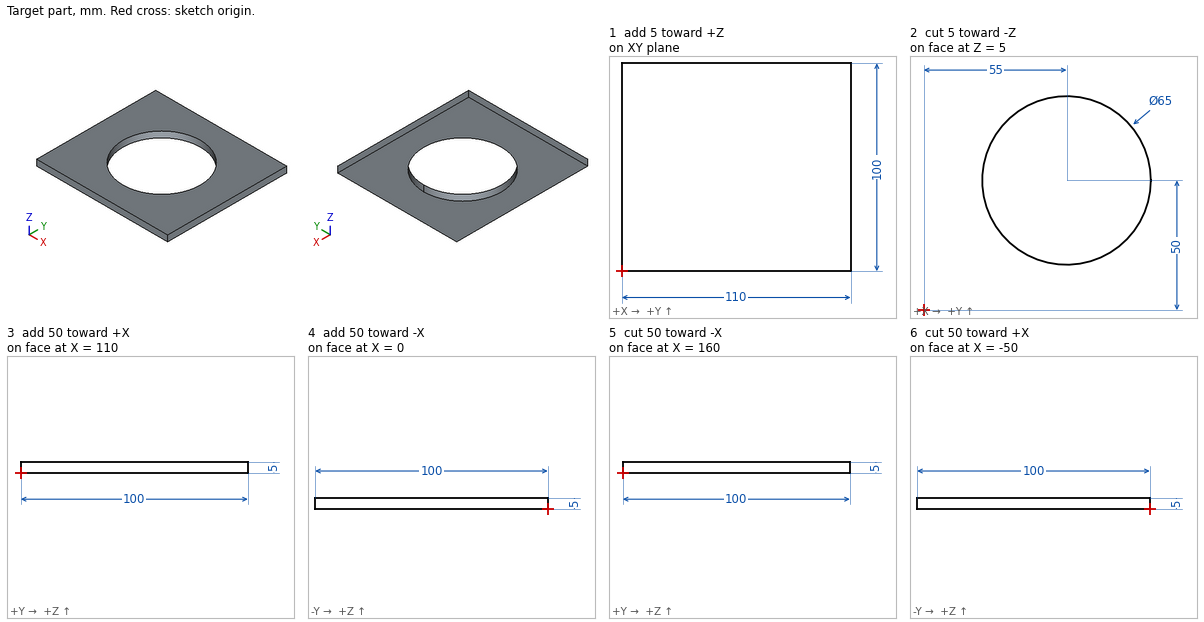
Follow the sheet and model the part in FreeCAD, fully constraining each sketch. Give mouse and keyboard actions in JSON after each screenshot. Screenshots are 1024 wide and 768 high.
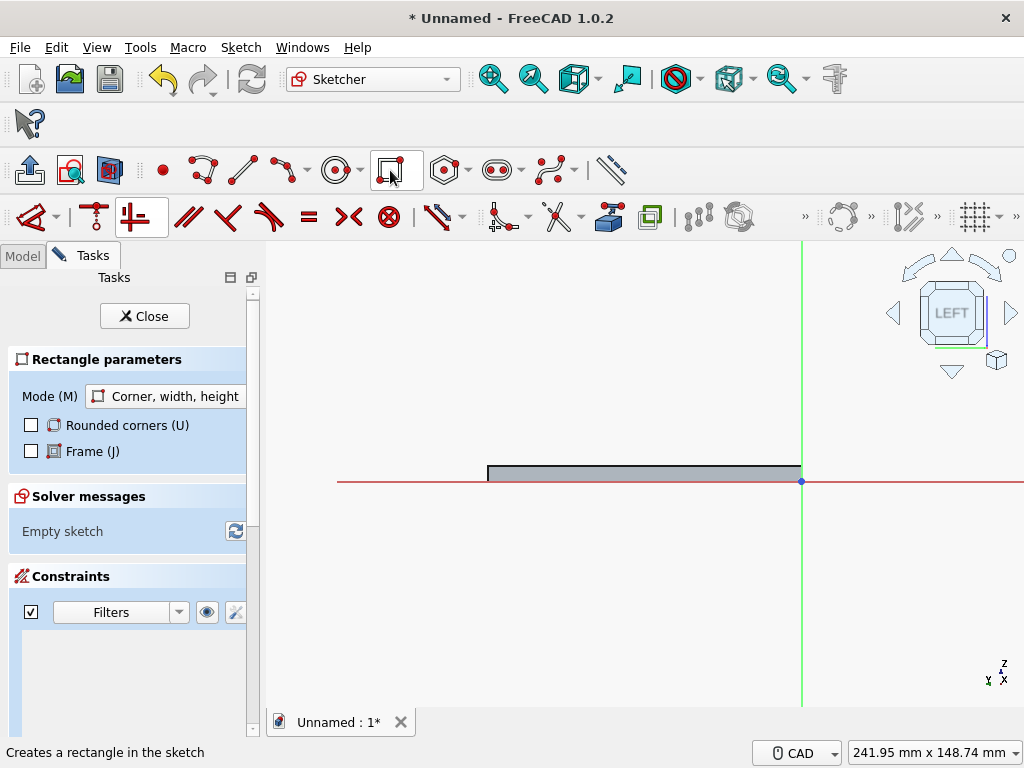
{"action": "left_click", "coordinate": [802, 482]}
{"action": "left_click", "coordinate": [488, 466]}
{"action": "key", "text": "Escape"}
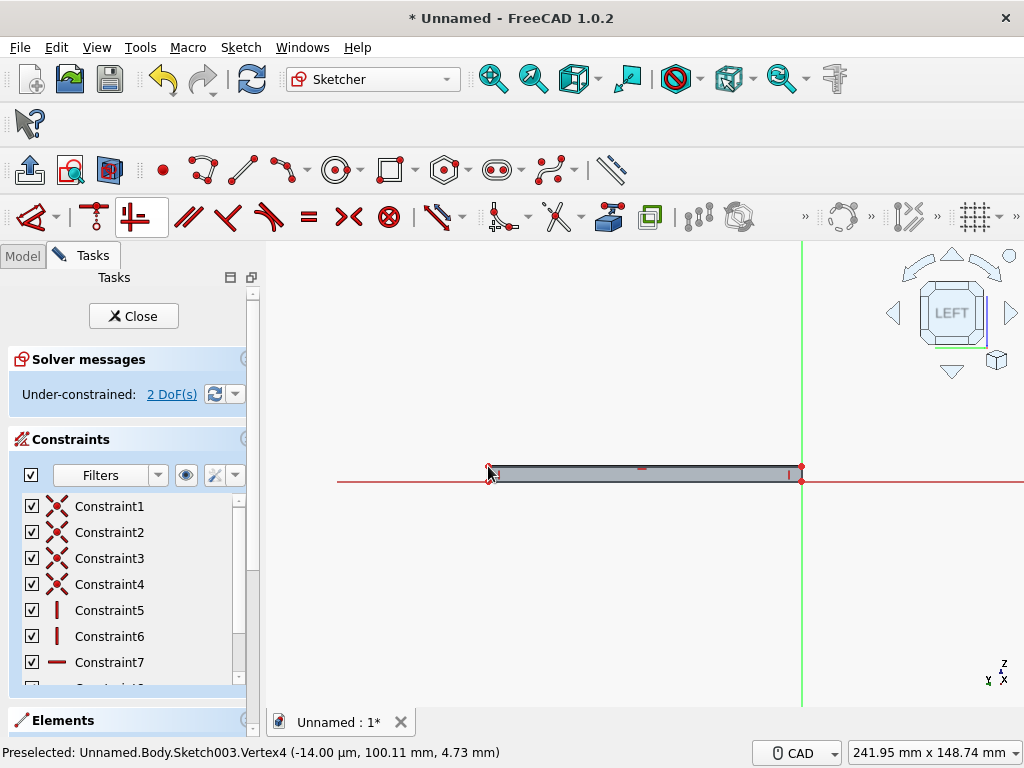
{"action": "left_click", "coordinate": [32, 218]}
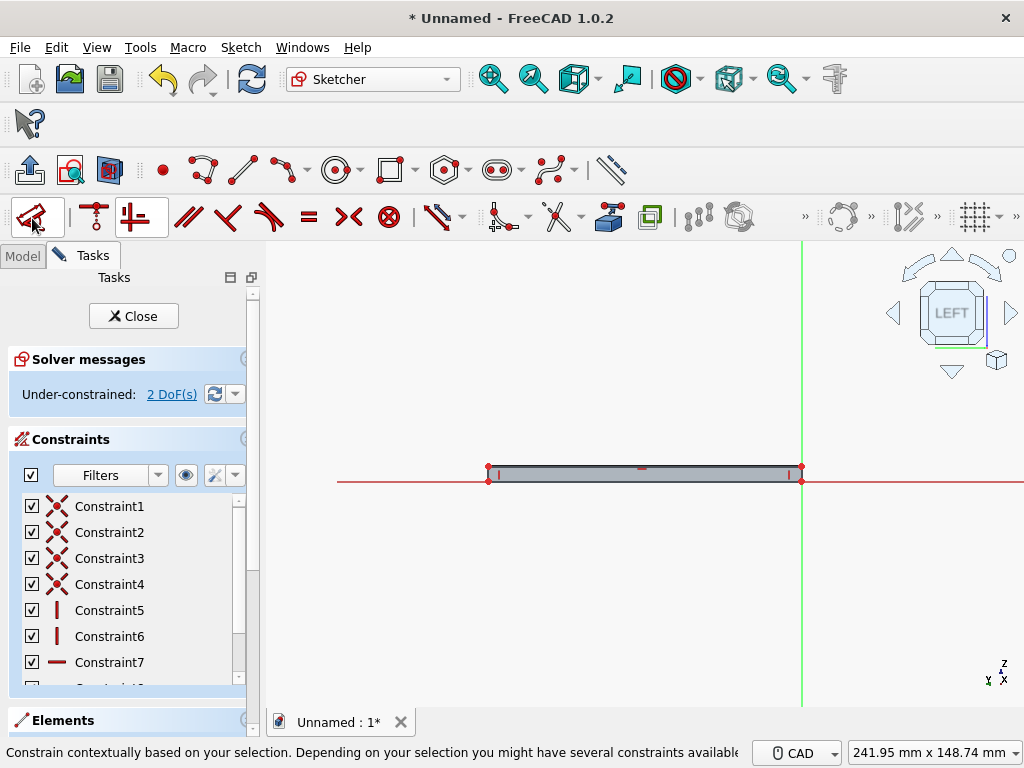
{"action": "scroll", "coordinate": [802, 474], "scroll_direction": "up", "scroll_amount": 5}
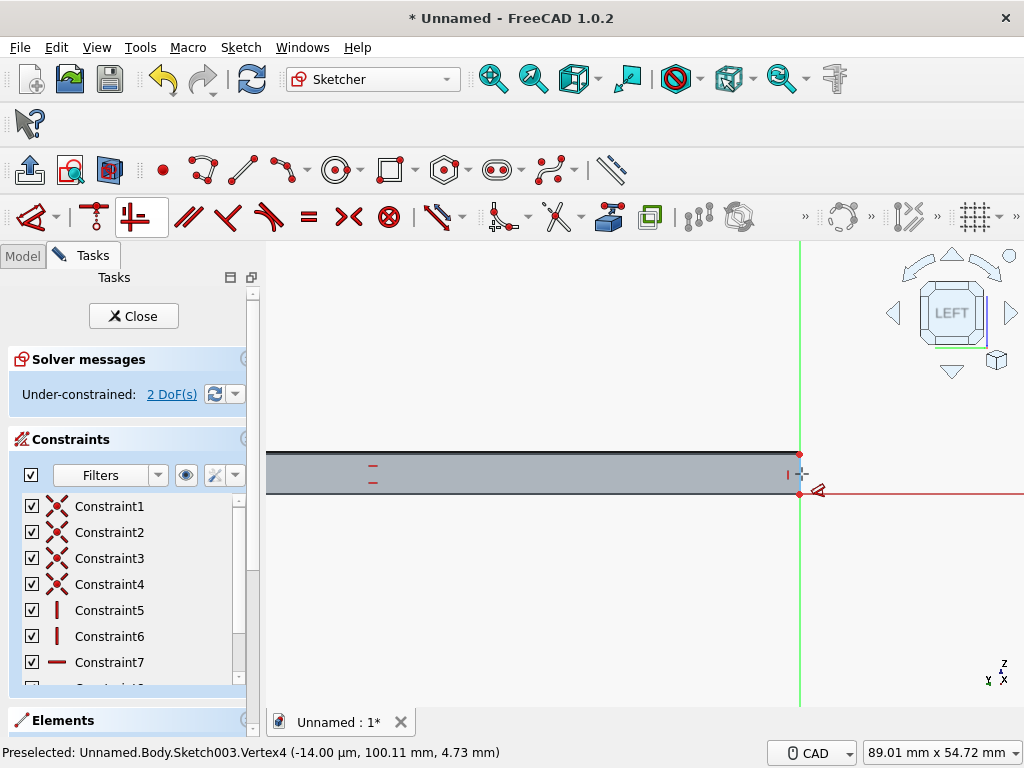
{"action": "left_click", "coordinate": [800, 474]}
{"action": "left_click", "coordinate": [834, 474]}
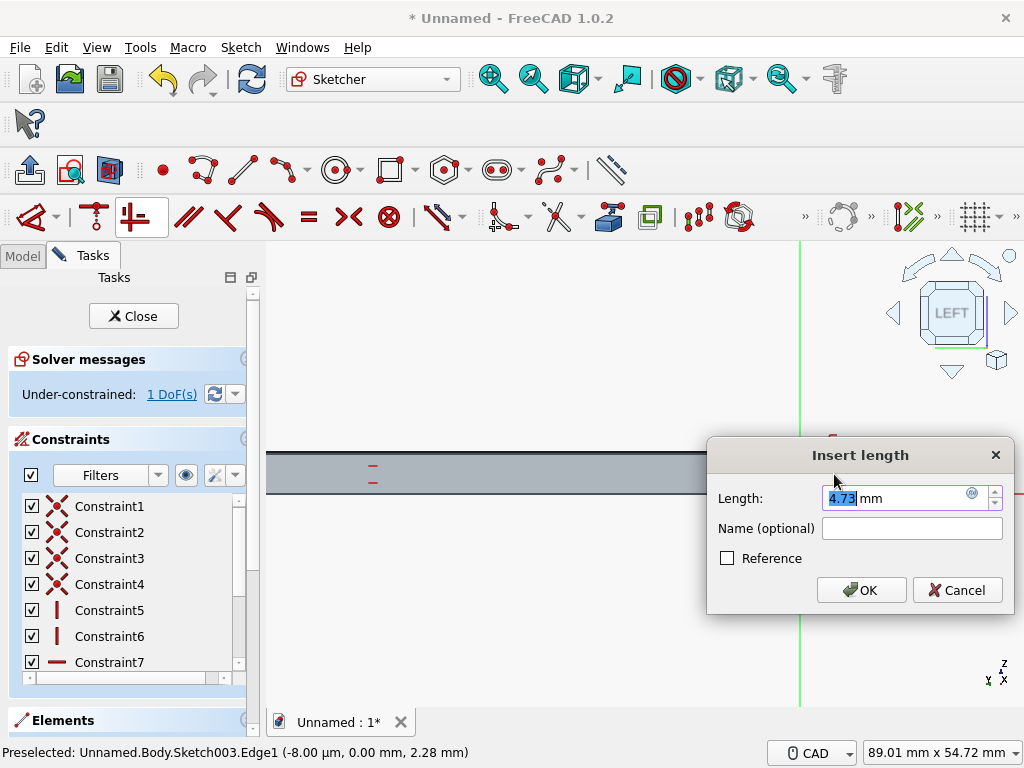
{"action": "type", "text": "5"}
{"action": "key", "text": "Return"}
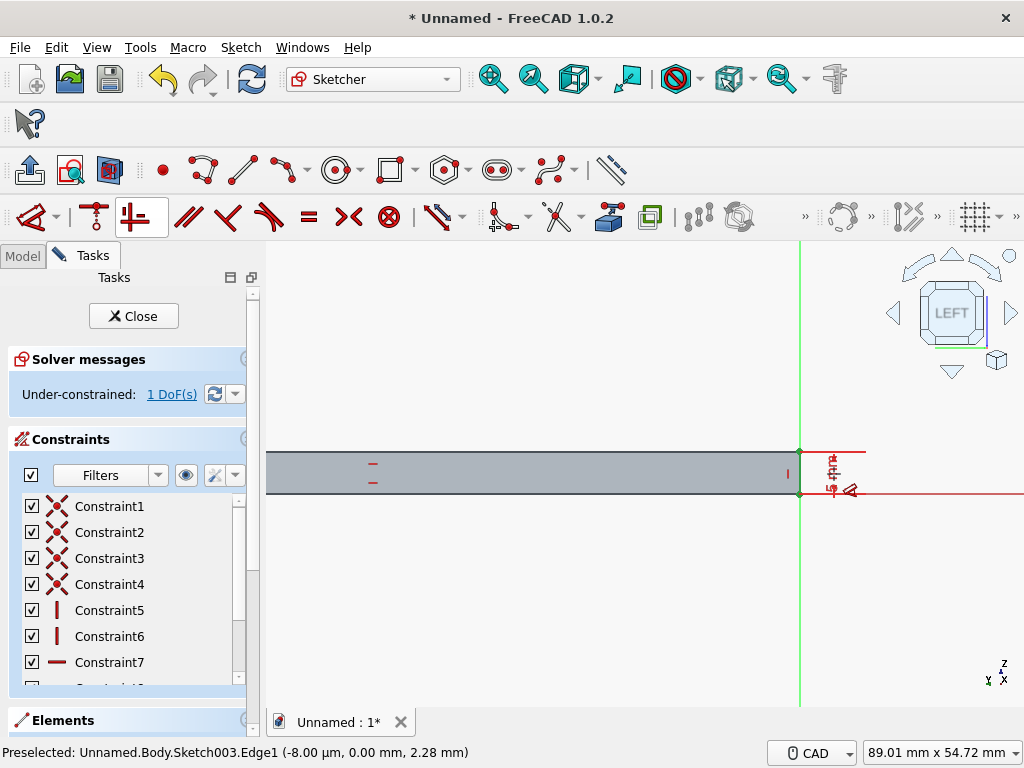
{"action": "left_click", "coordinate": [544, 452]}
{"action": "left_click", "coordinate": [547, 418]}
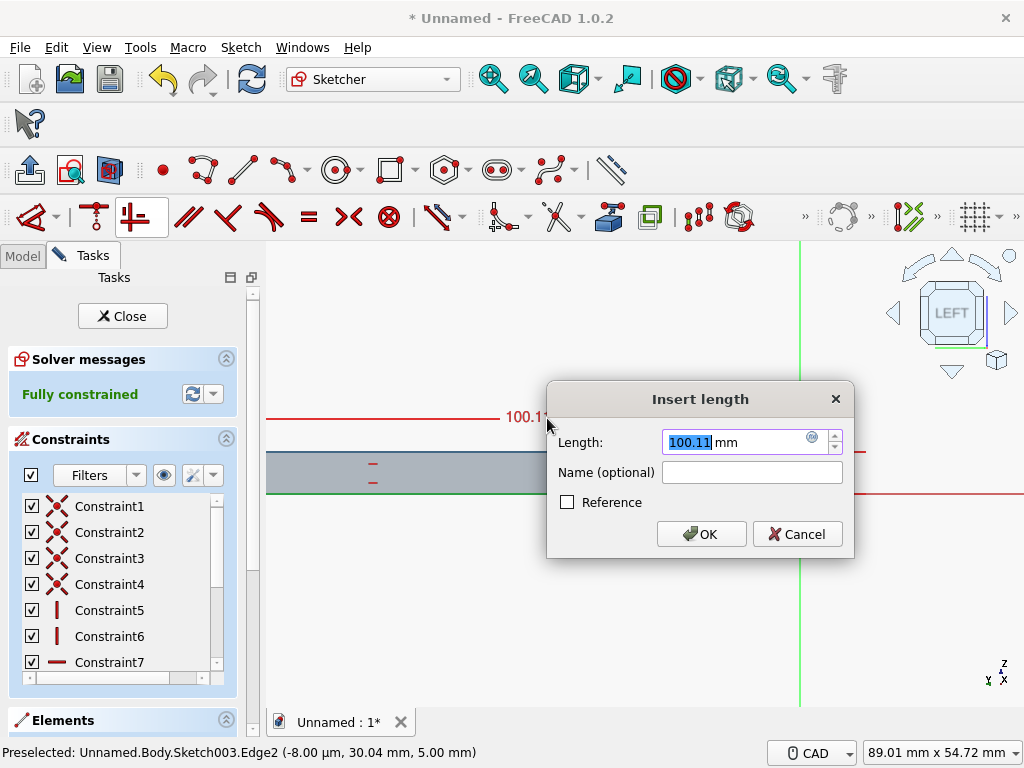
{"action": "type", "text": "100"}
{"action": "key", "text": "Return"}
{"action": "key", "text": "Escape"}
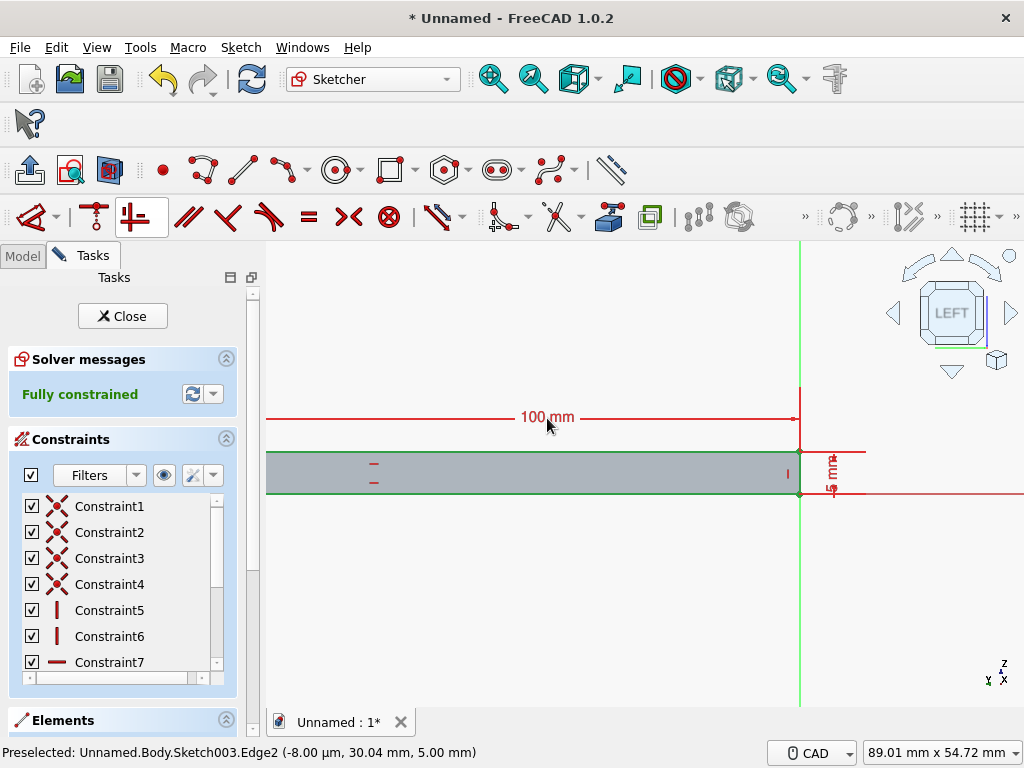
{"action": "left_click", "coordinate": [123, 316]}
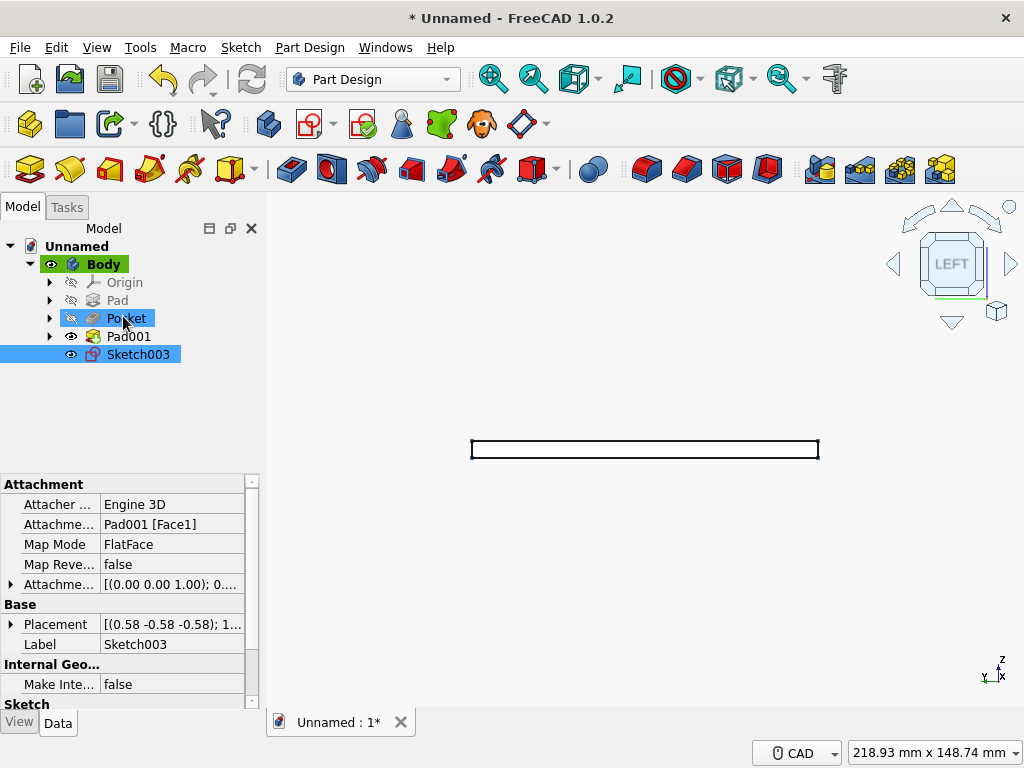
{"action": "left_click", "coordinate": [30, 170]}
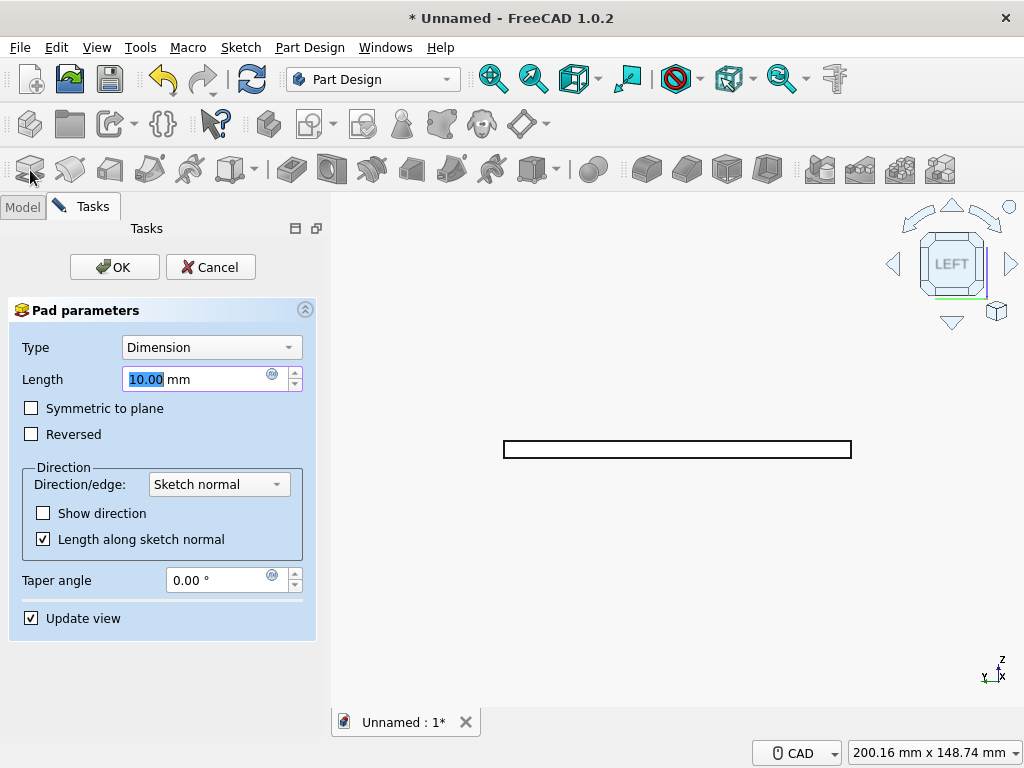
{"action": "type", "text": "50"}
{"action": "key", "text": "Tab"}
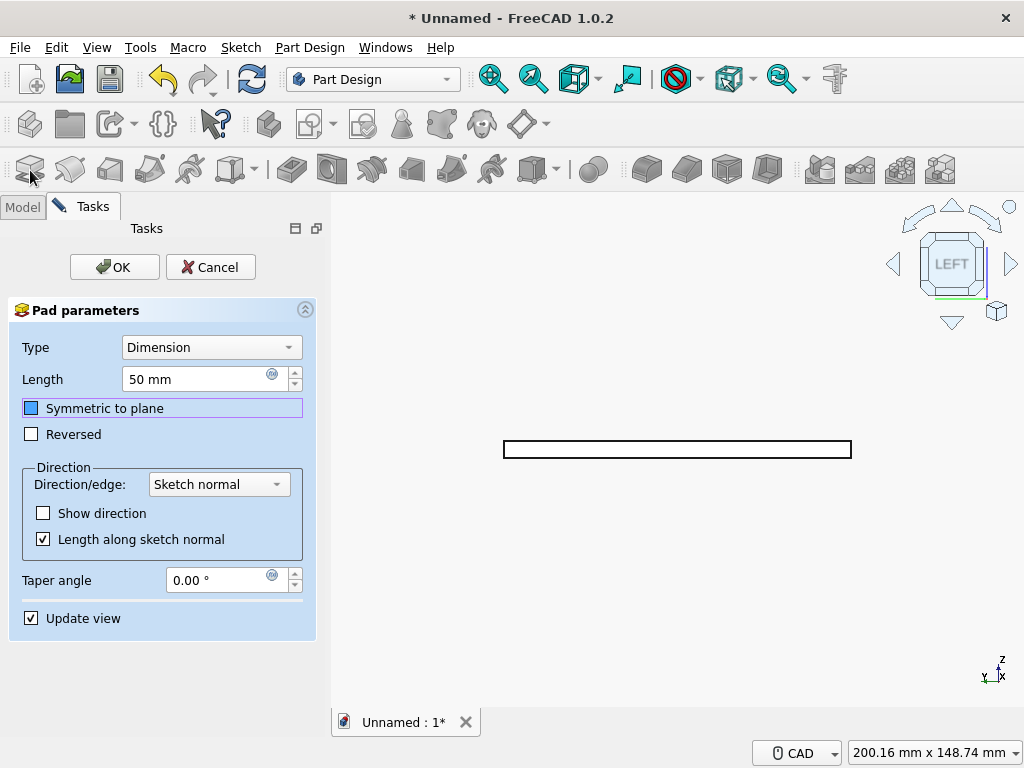
{"action": "left_click", "coordinate": [115, 267]}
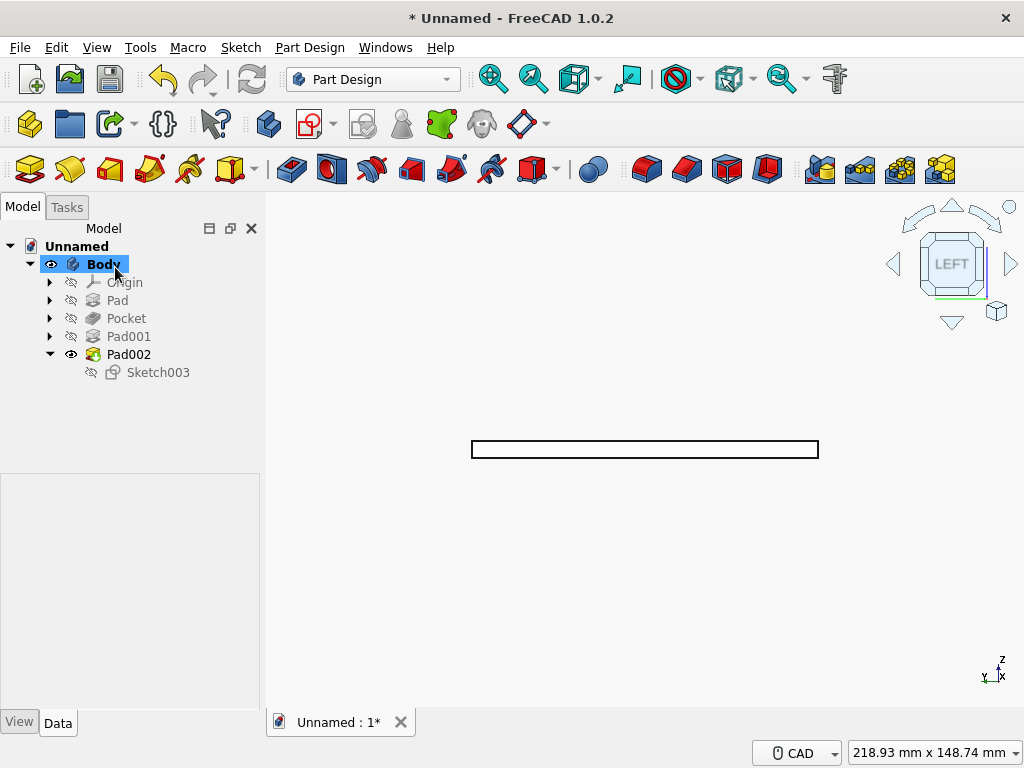
{"action": "key", "text": "0"}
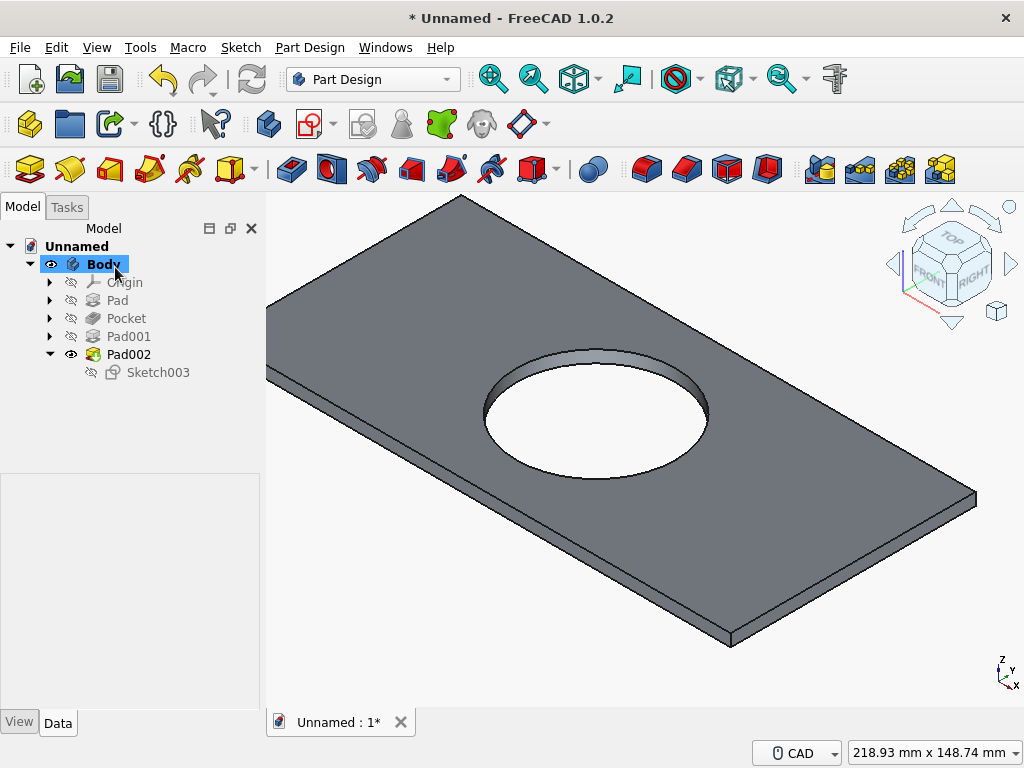
{"action": "left_click", "coordinate": [494, 80]}